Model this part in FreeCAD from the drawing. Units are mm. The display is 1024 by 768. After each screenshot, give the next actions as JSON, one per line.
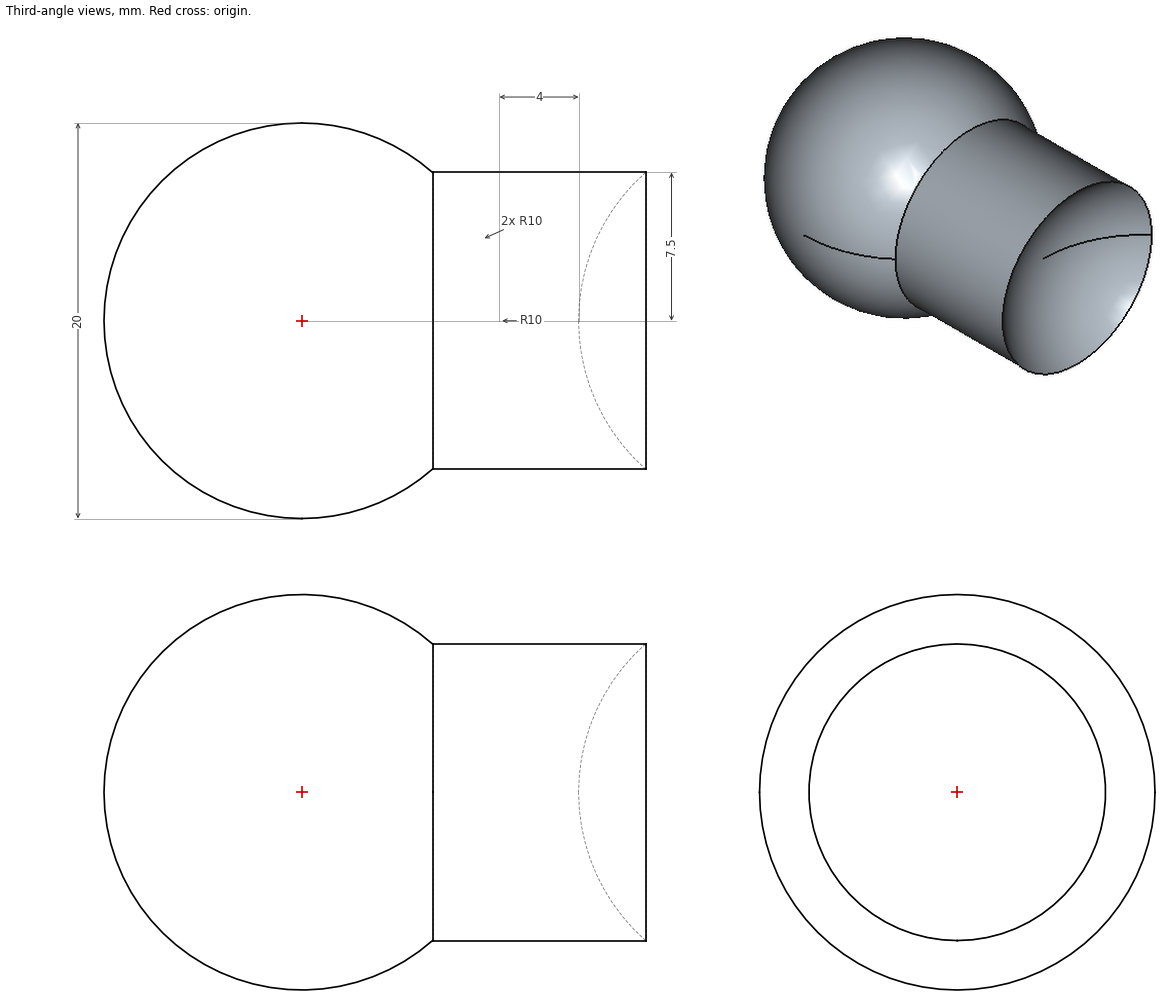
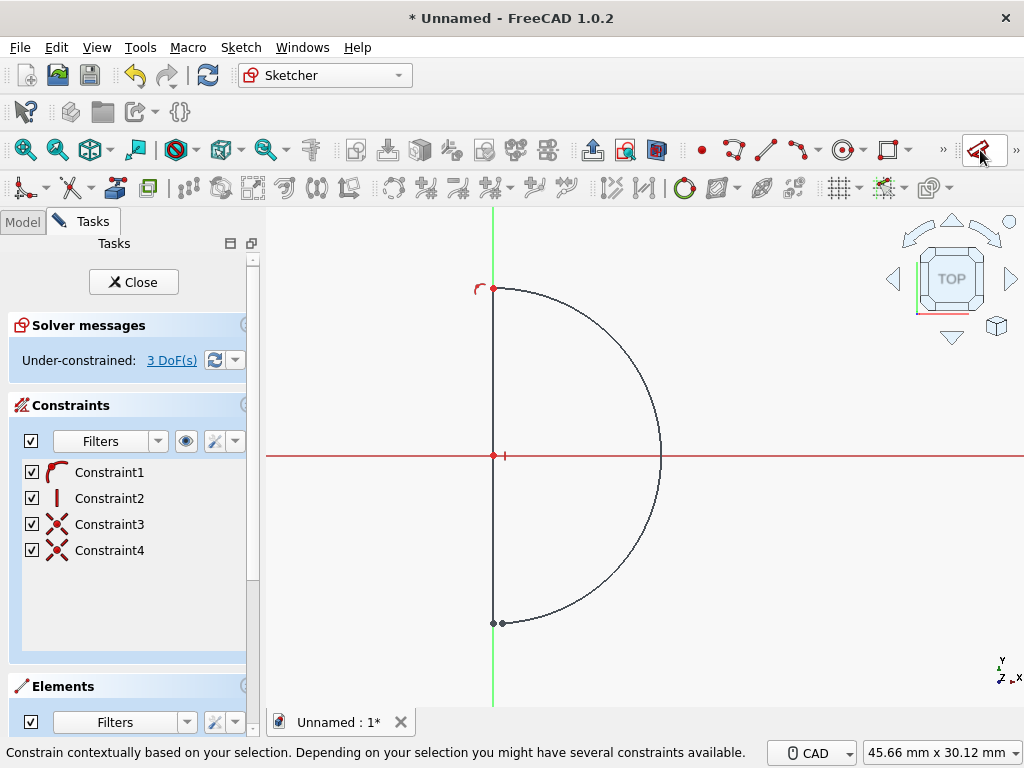
{"action": "left_click", "coordinate": [633, 549]}
{"action": "left_click", "coordinate": [660, 567]}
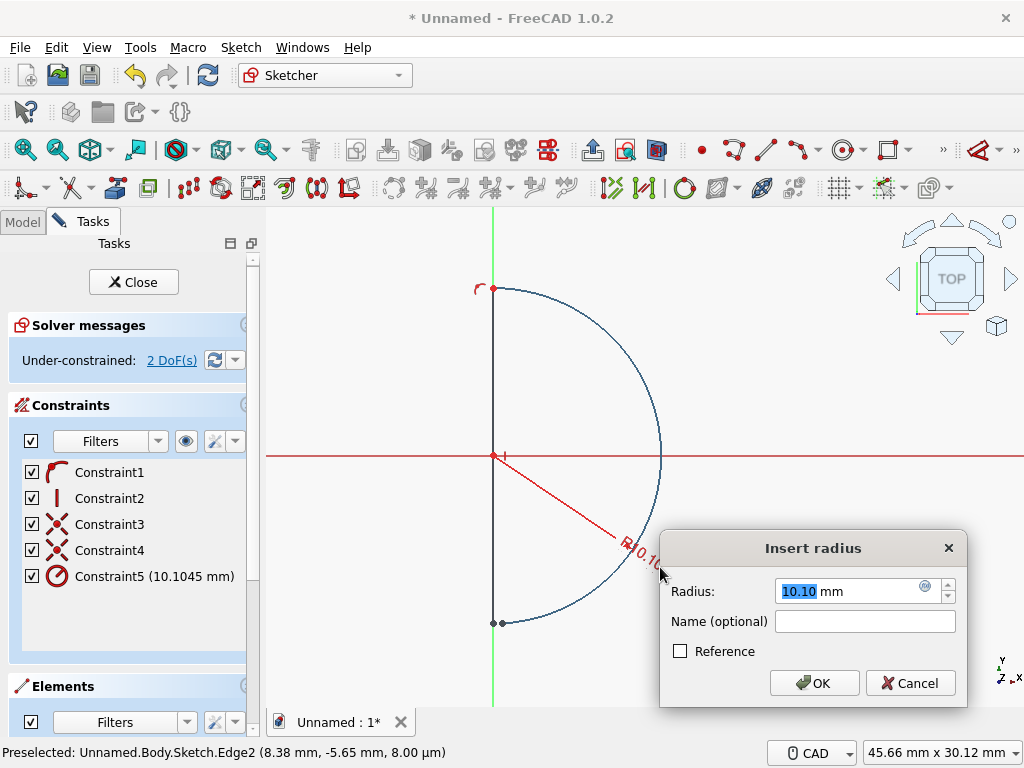
{"action": "type", "text": "10"}
{"action": "key", "text": "Return"}
{"action": "key", "text": "Escape"}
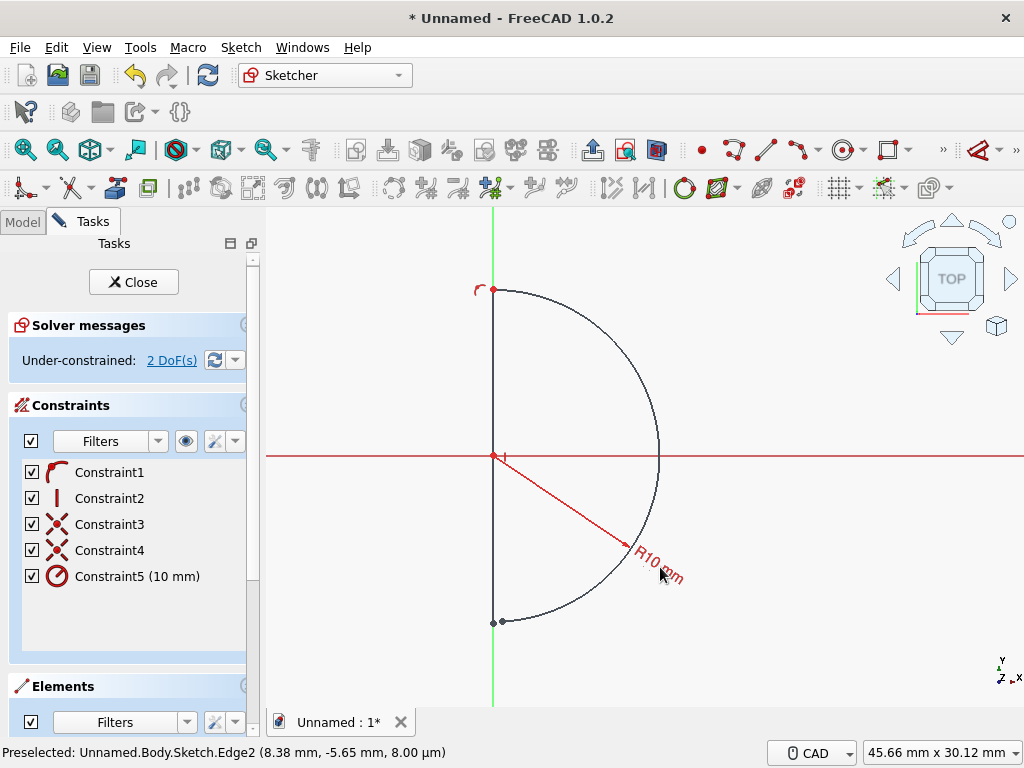
{"action": "left_click", "coordinate": [503, 622]}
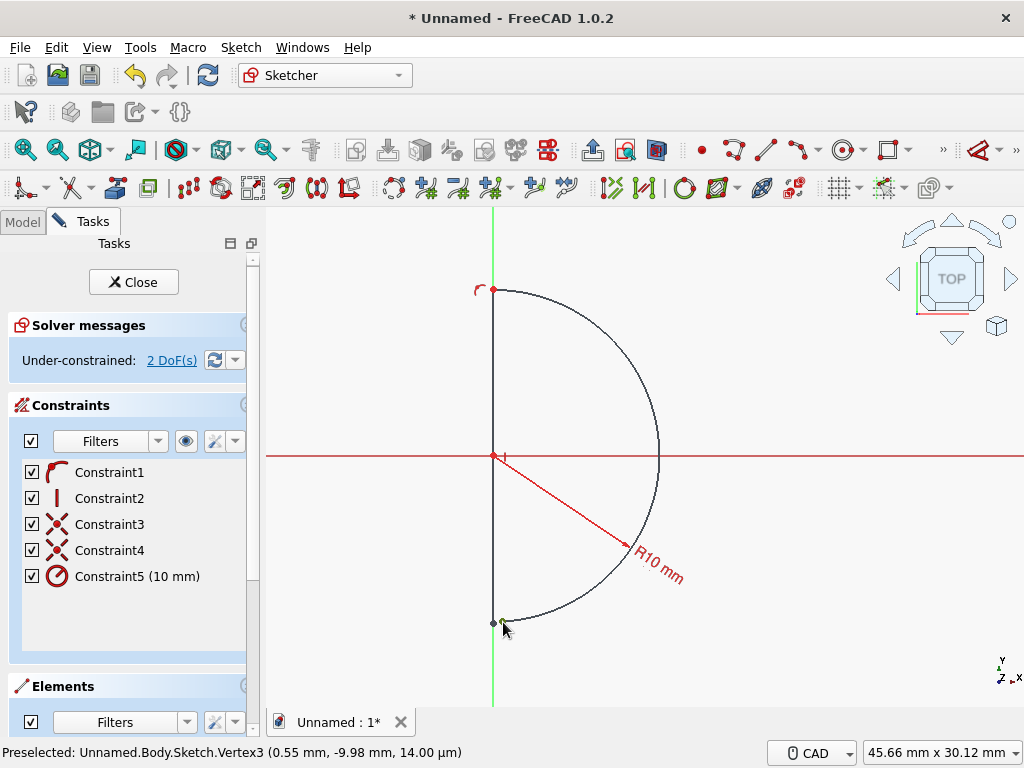
{"action": "left_click", "coordinate": [493, 647]}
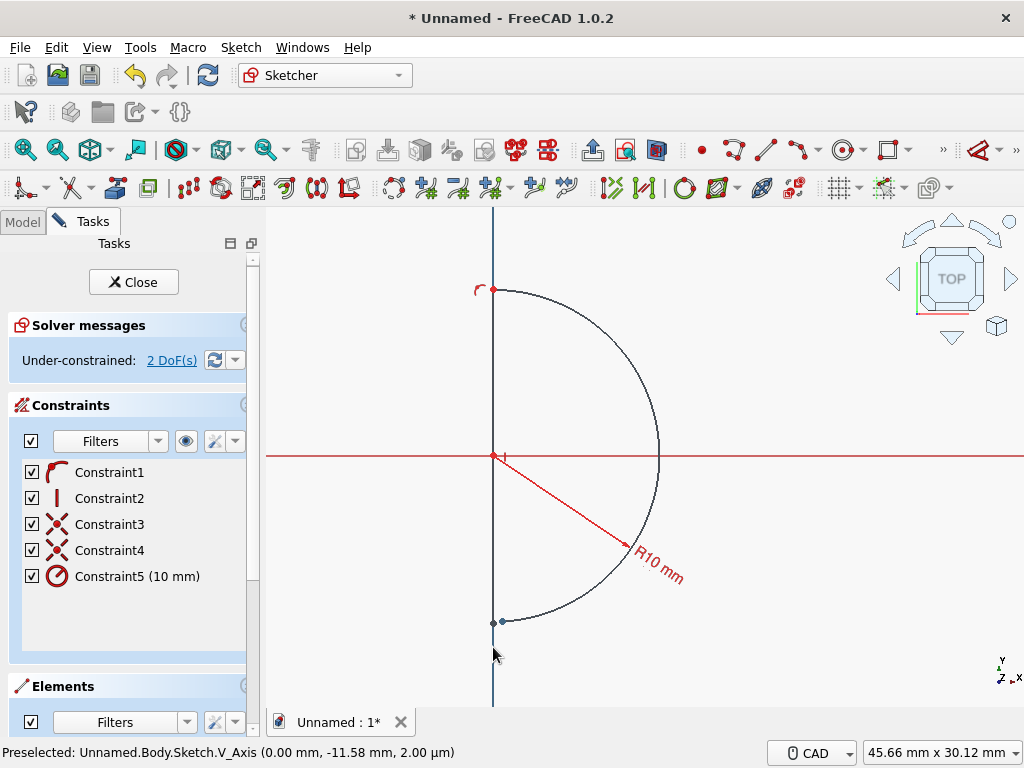
{"action": "key", "text": "c"}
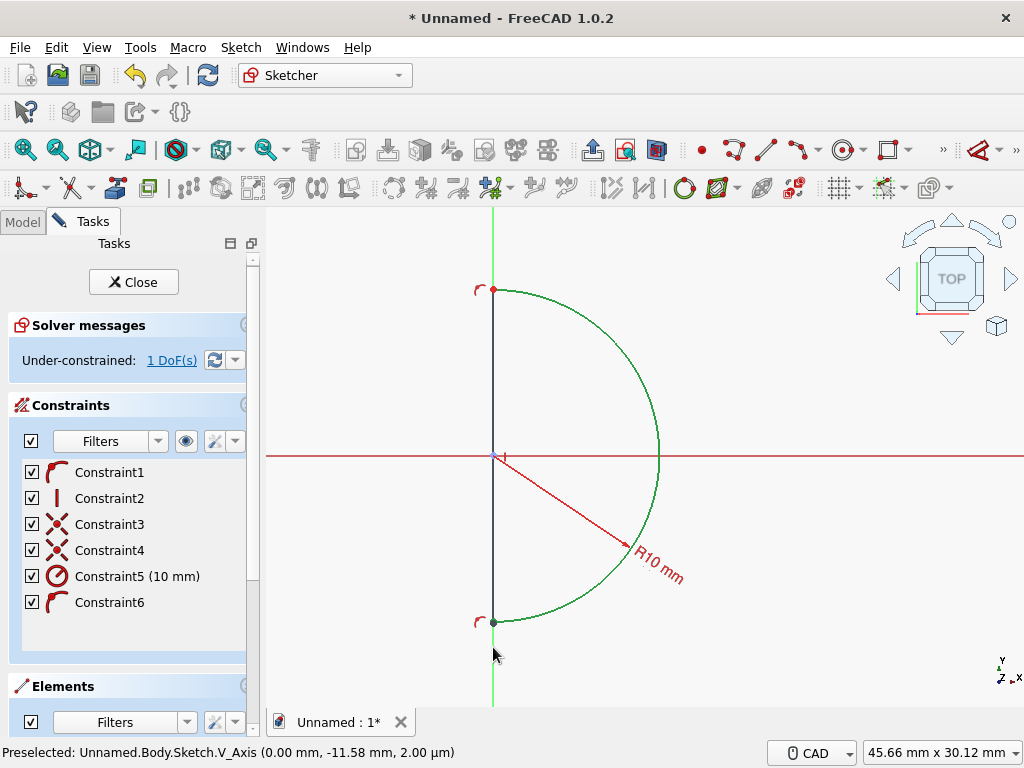
{"action": "key", "text": "d"}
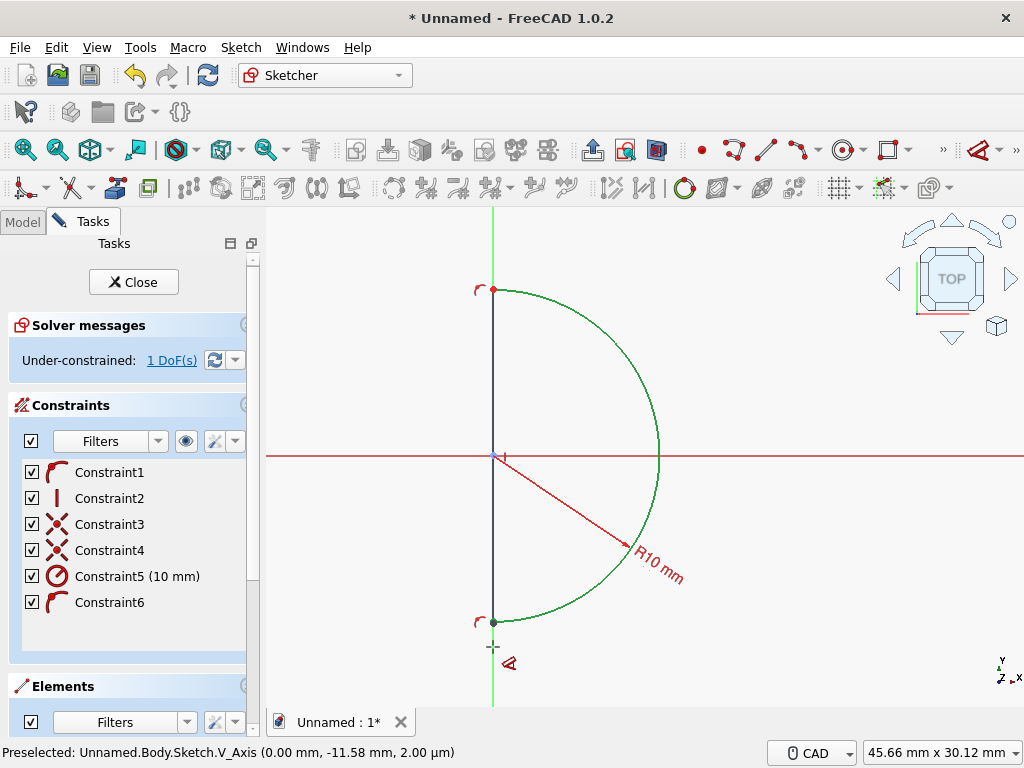
{"action": "left_click", "coordinate": [493, 390]}
{"action": "left_click", "coordinate": [459, 380]}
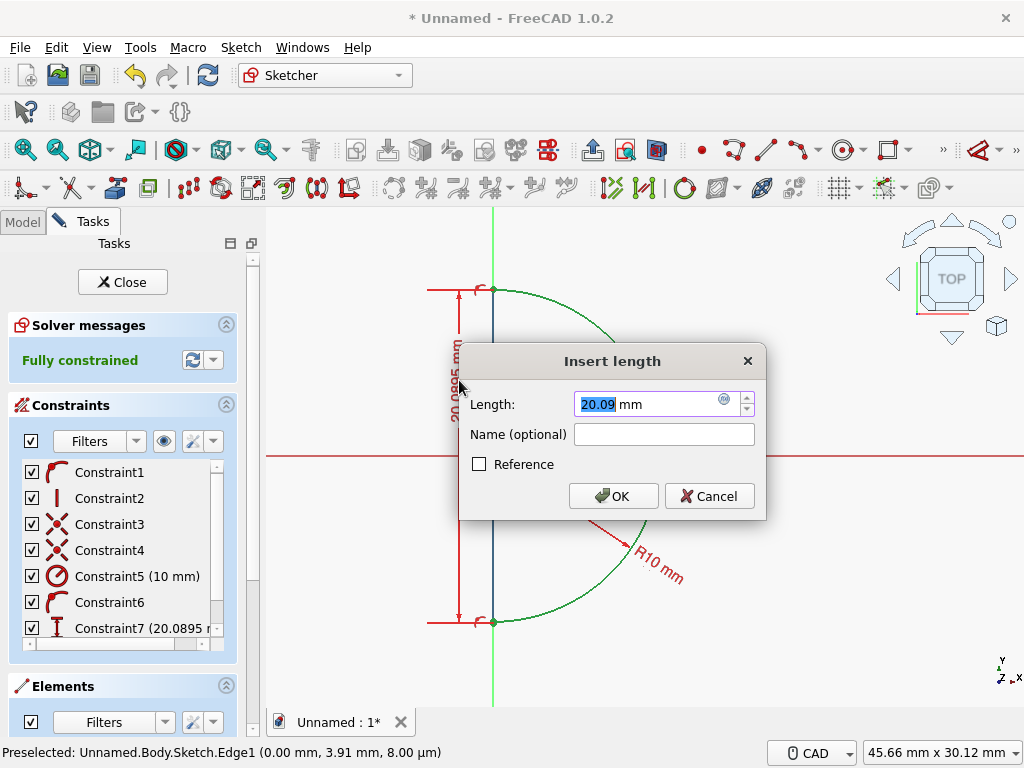
{"action": "type", "text": "20"}
{"action": "key", "text": "Return"}
{"action": "key", "text": "Escape"}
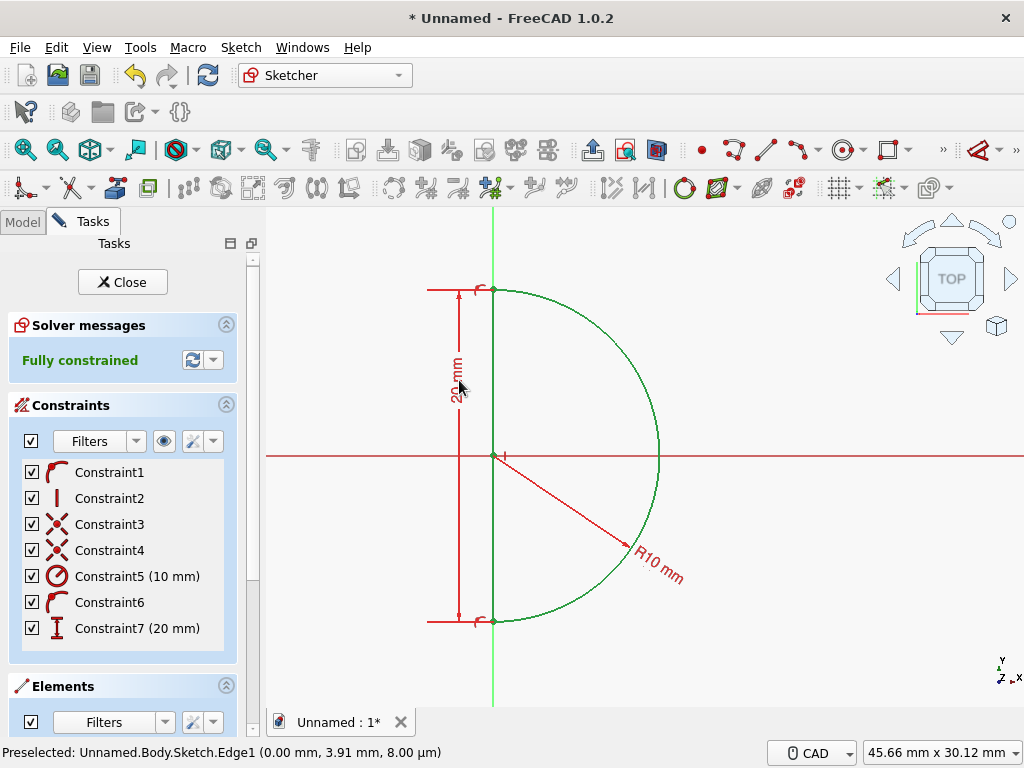
{"action": "left_click", "coordinate": [123, 282]}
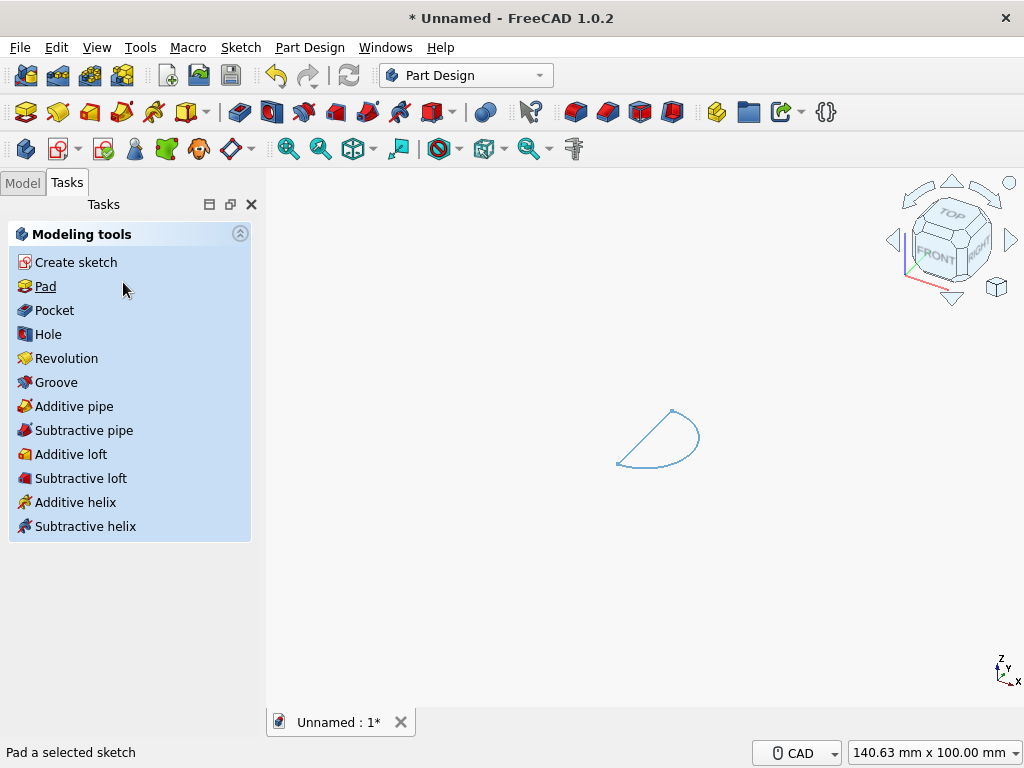
{"action": "left_click", "coordinate": [58, 112]}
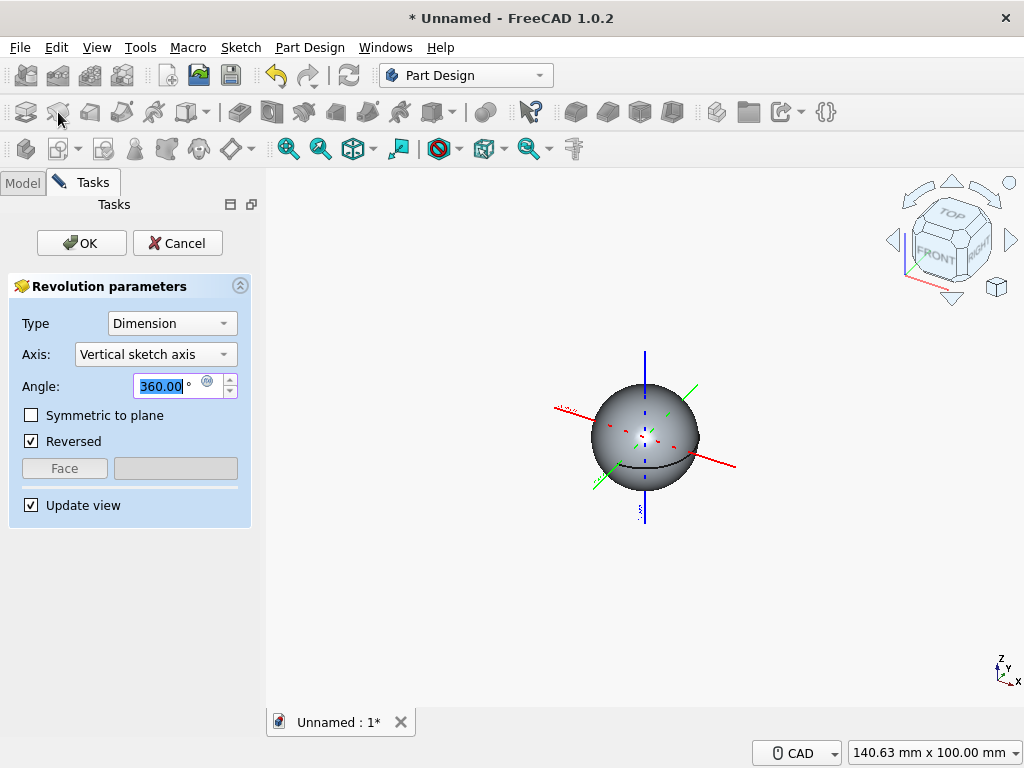
{"action": "left_click", "coordinate": [82, 243]}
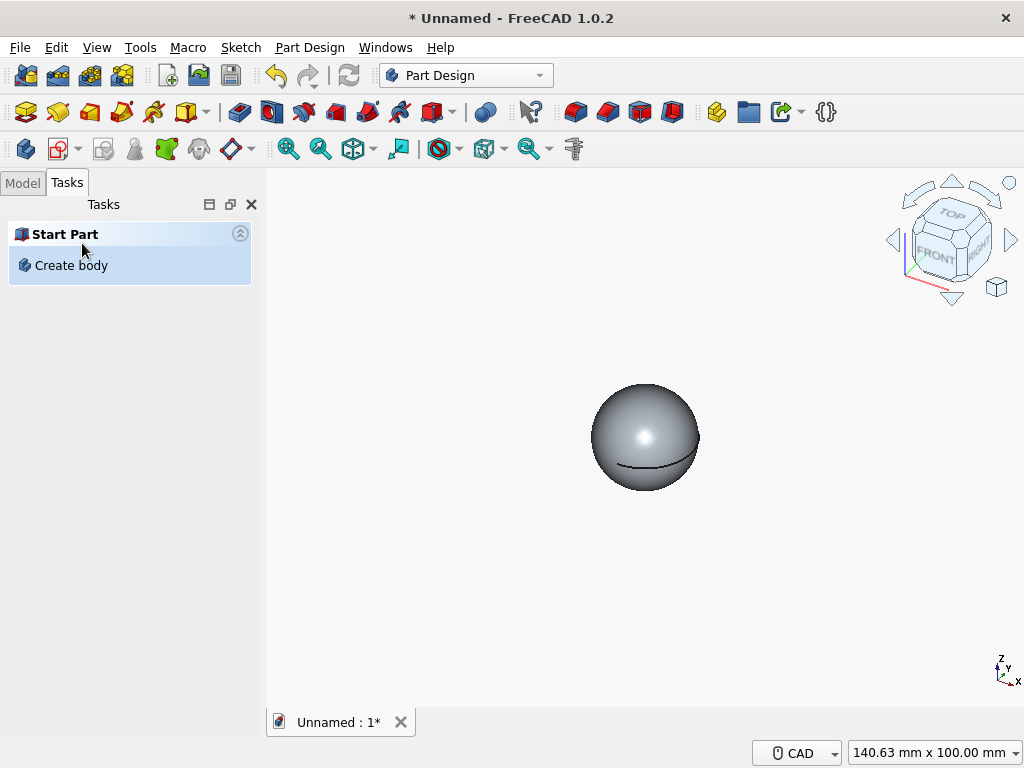
{"action": "left_click", "coordinate": [290, 150]}